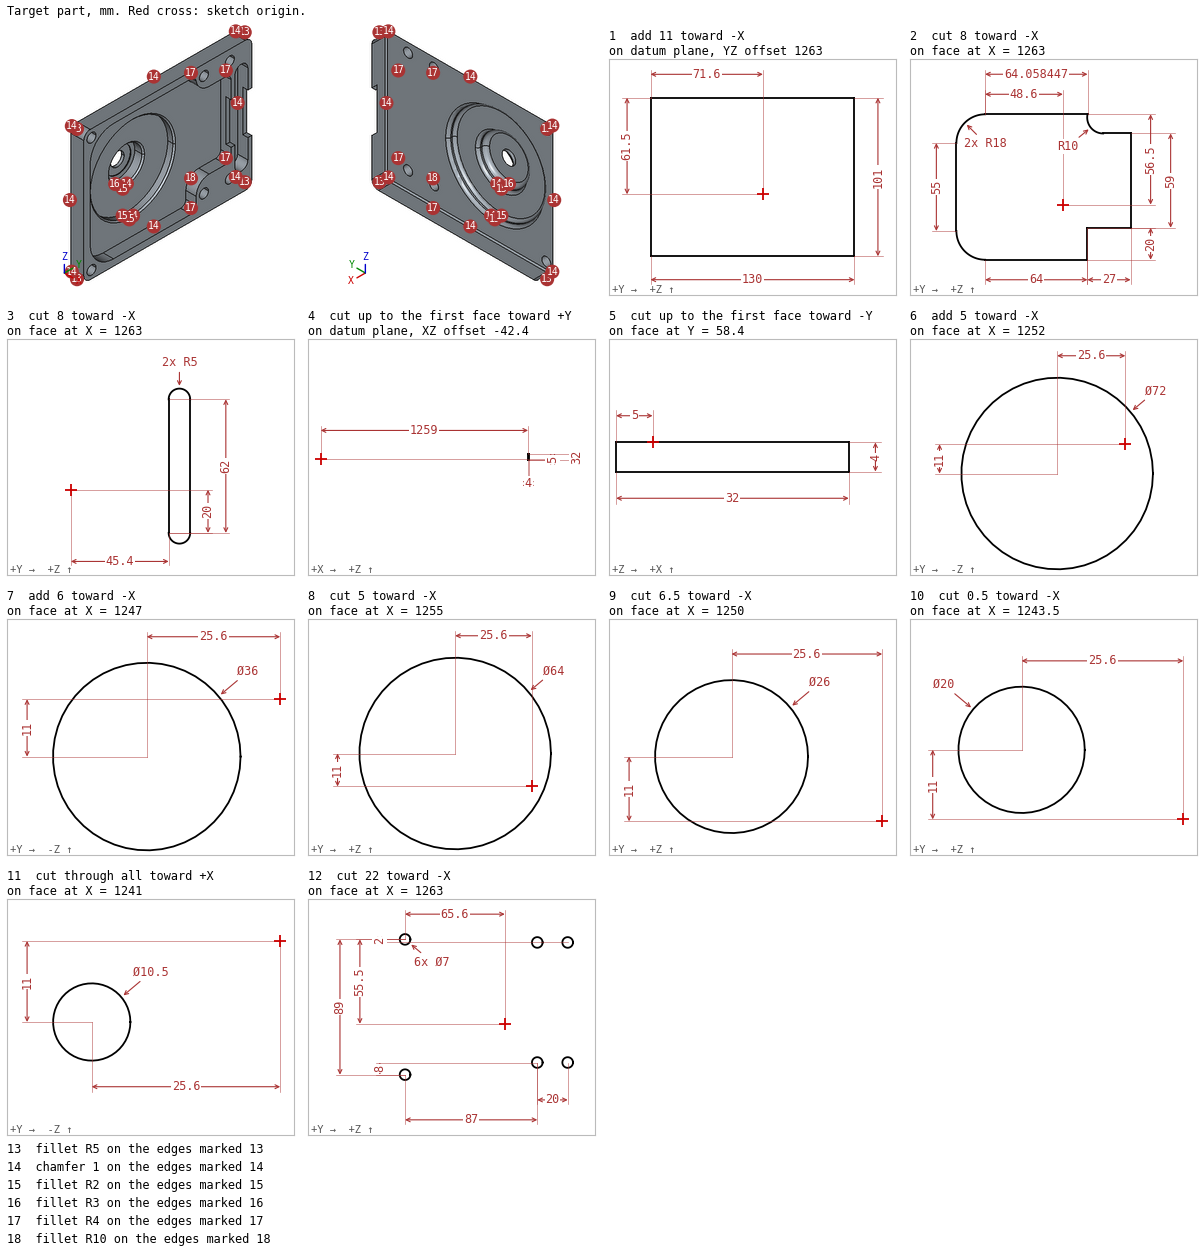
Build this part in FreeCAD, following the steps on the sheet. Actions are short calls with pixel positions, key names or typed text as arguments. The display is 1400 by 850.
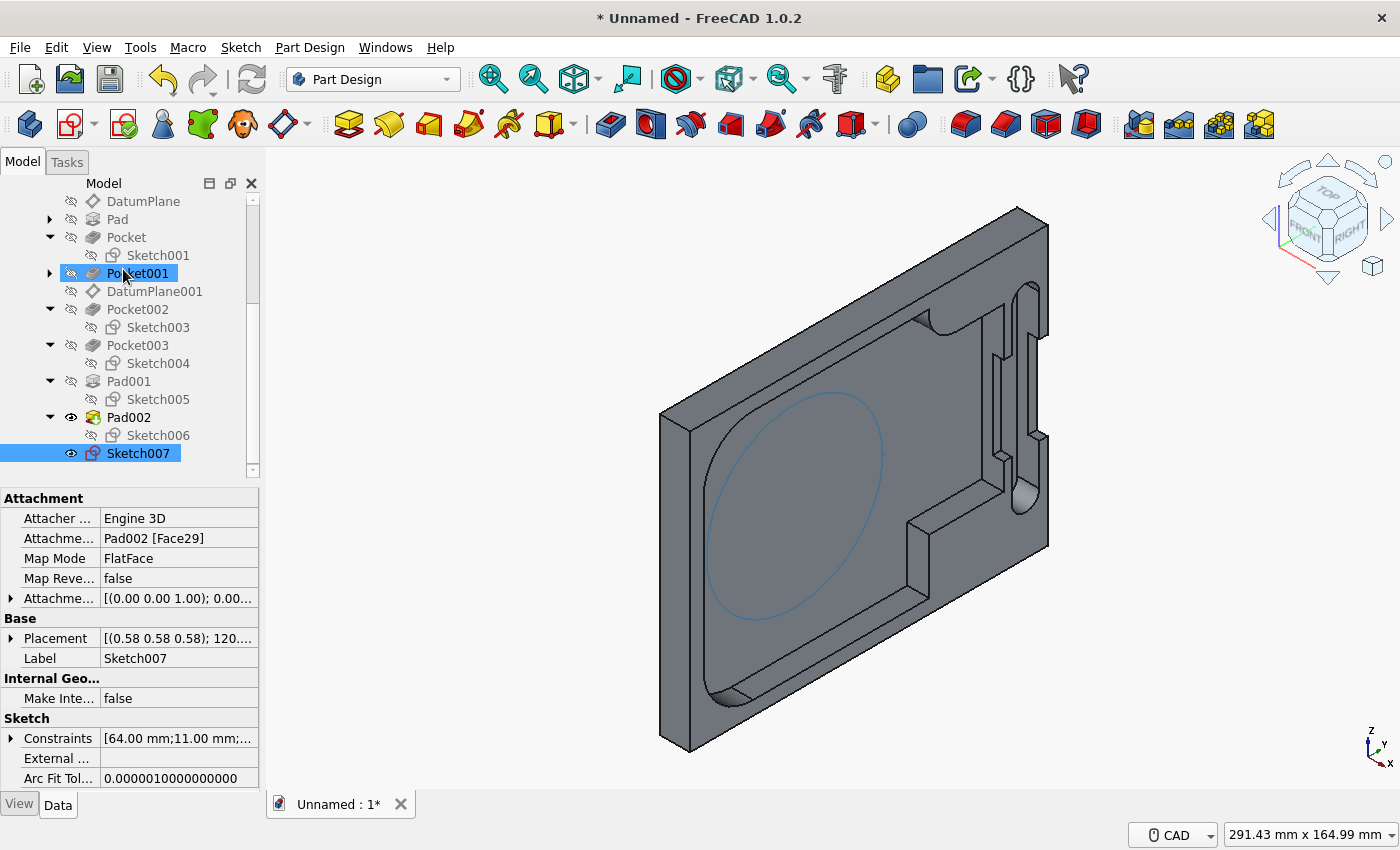
click(612, 124)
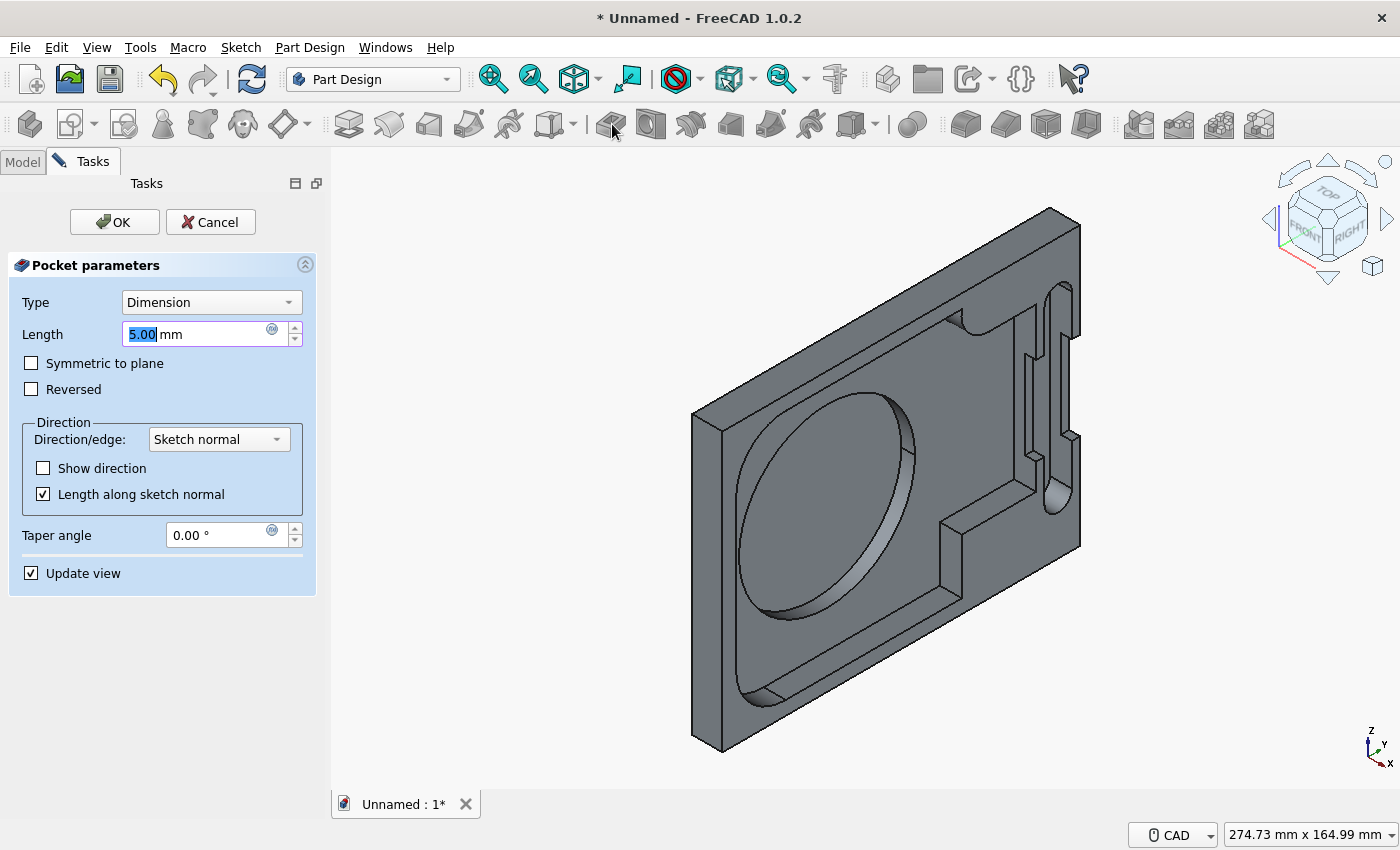
text(5)
key(Tab)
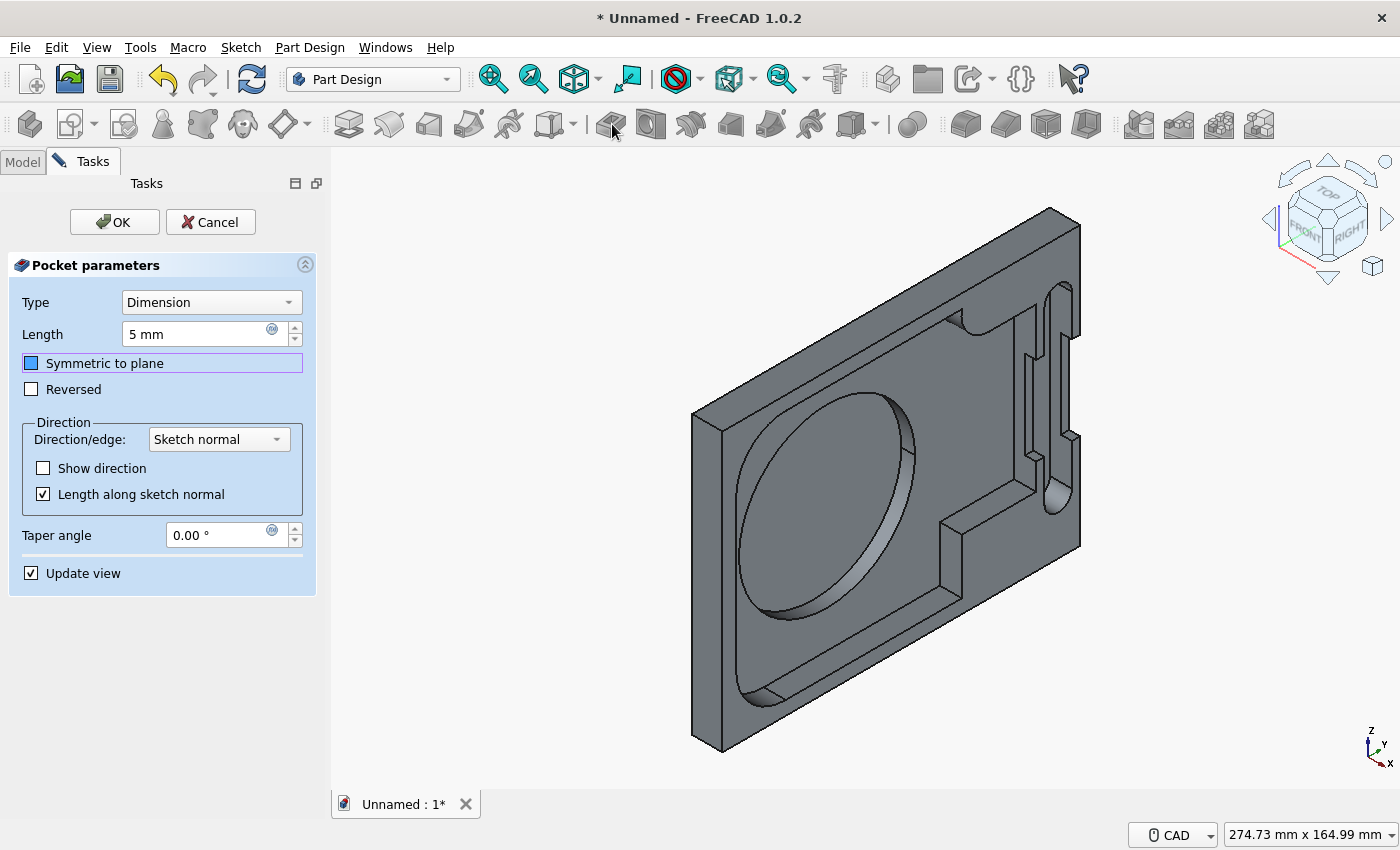
click(115, 222)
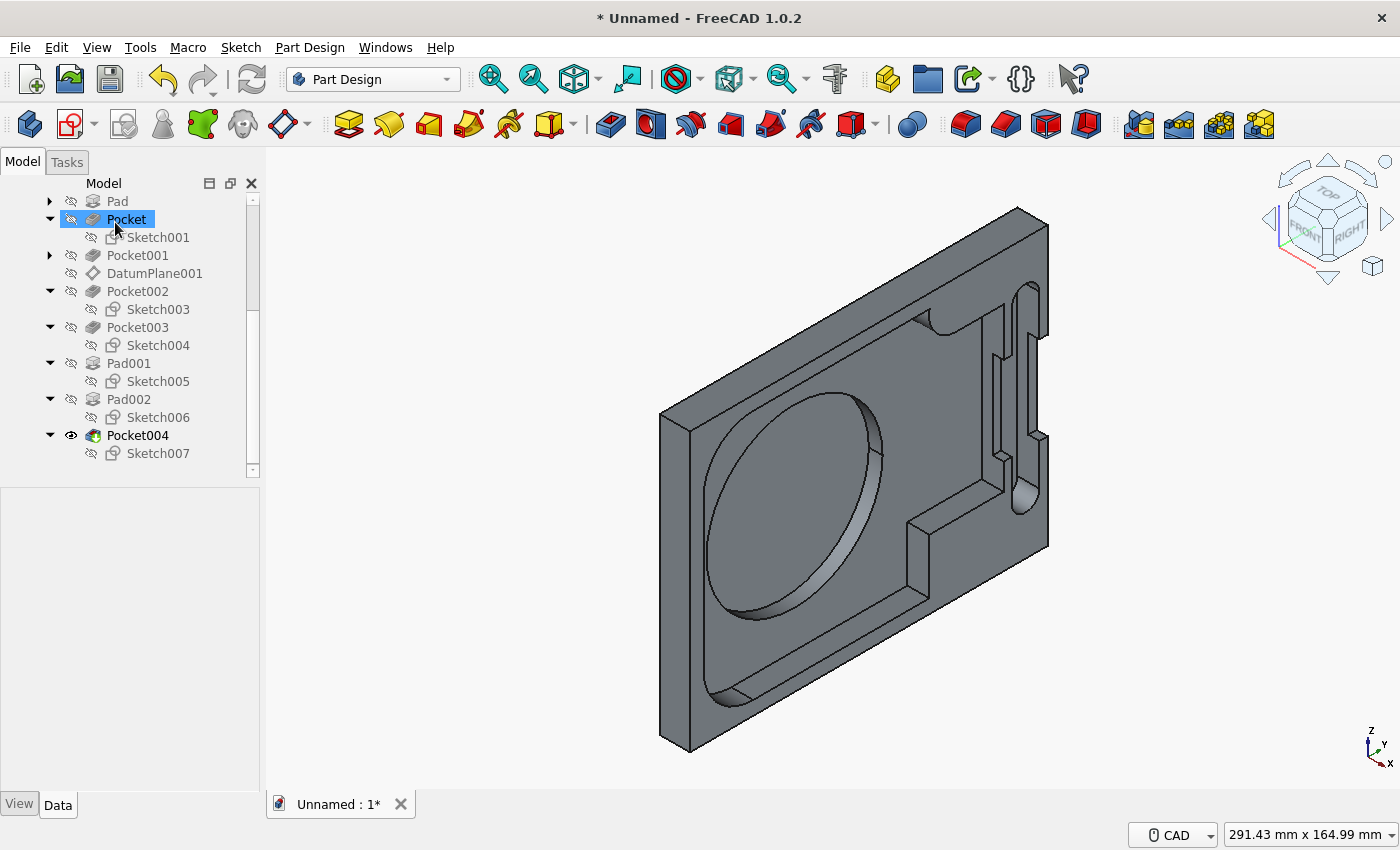
click(781, 497)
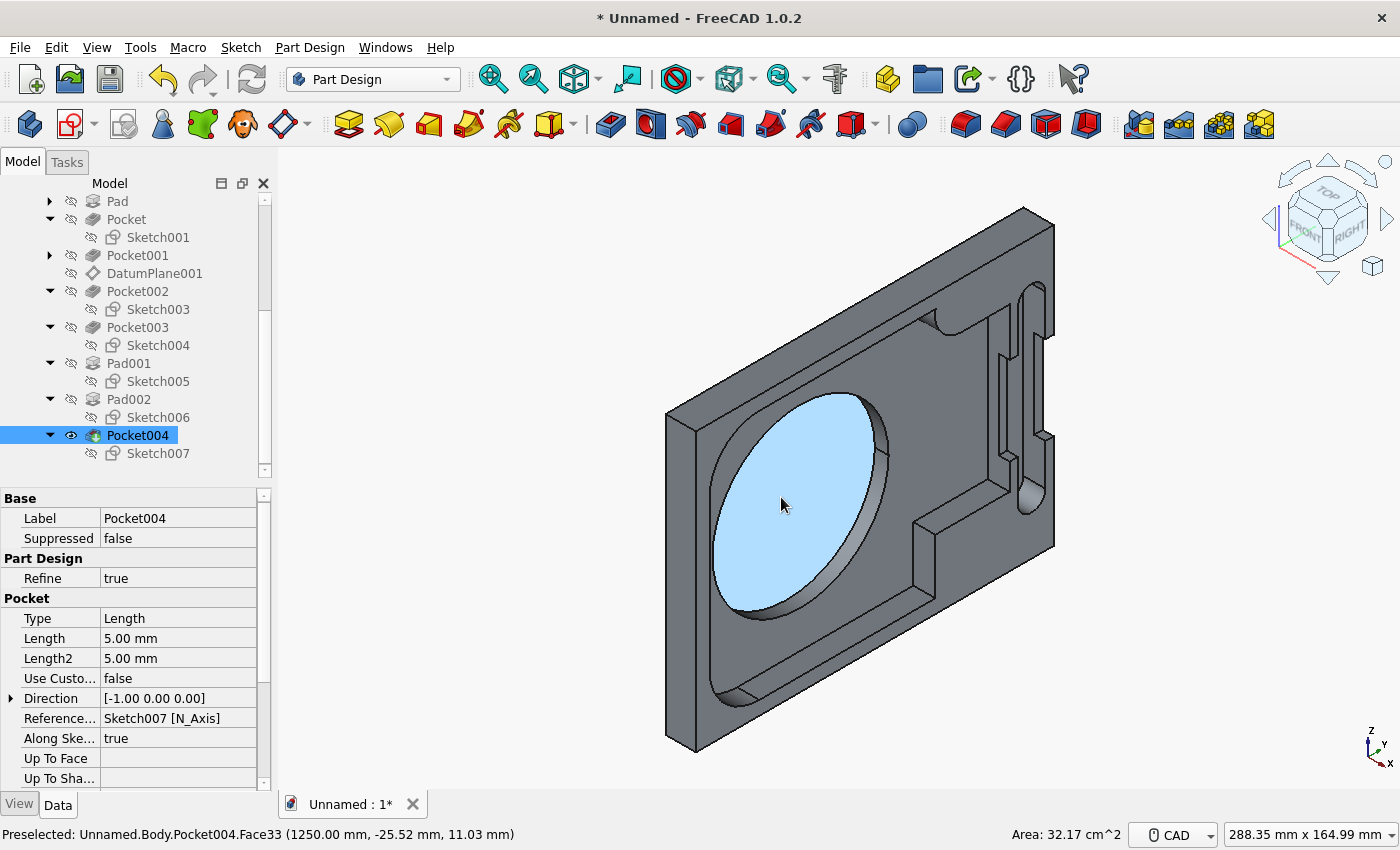
click(70, 124)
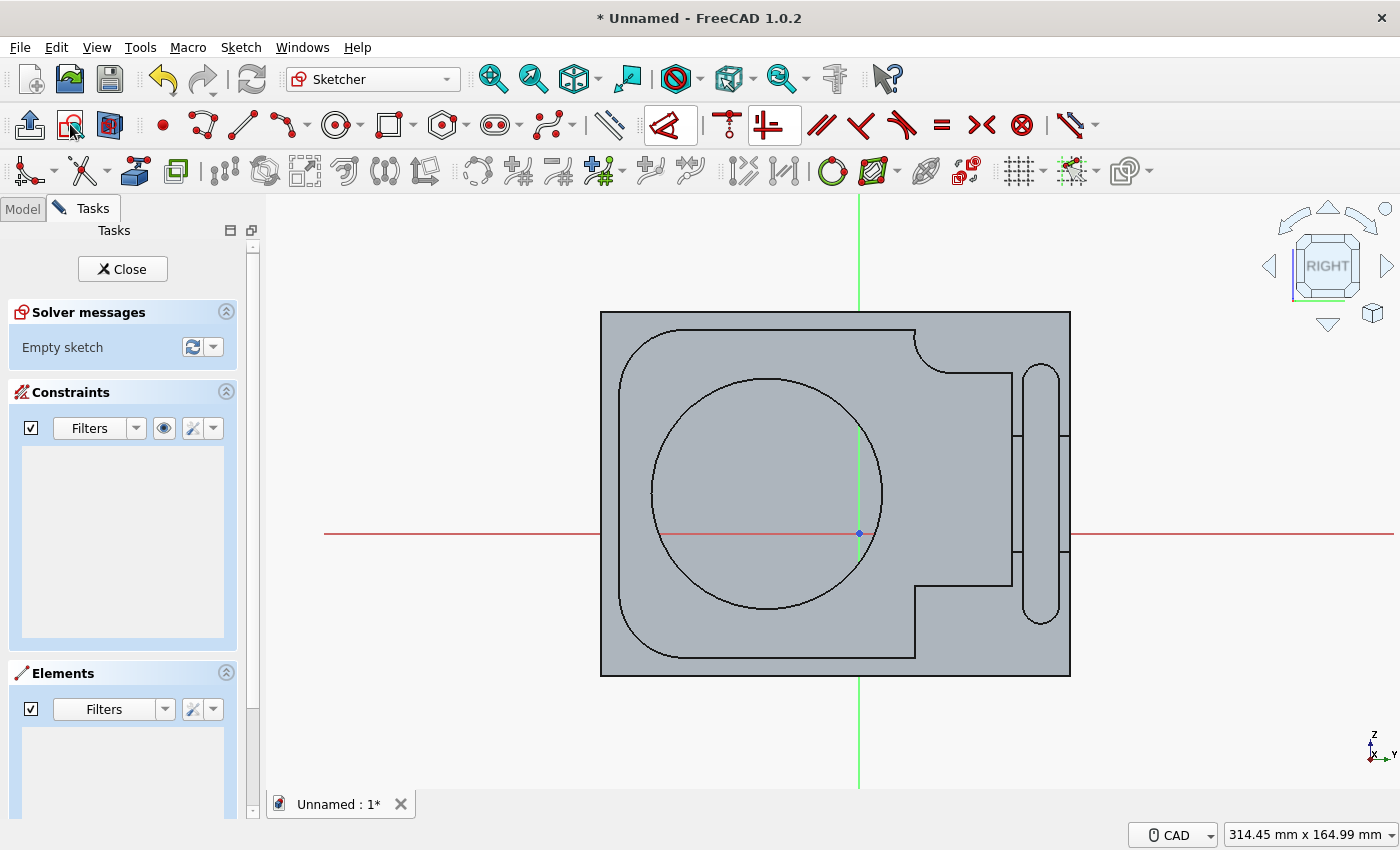
scroll(798, 495, up, 7)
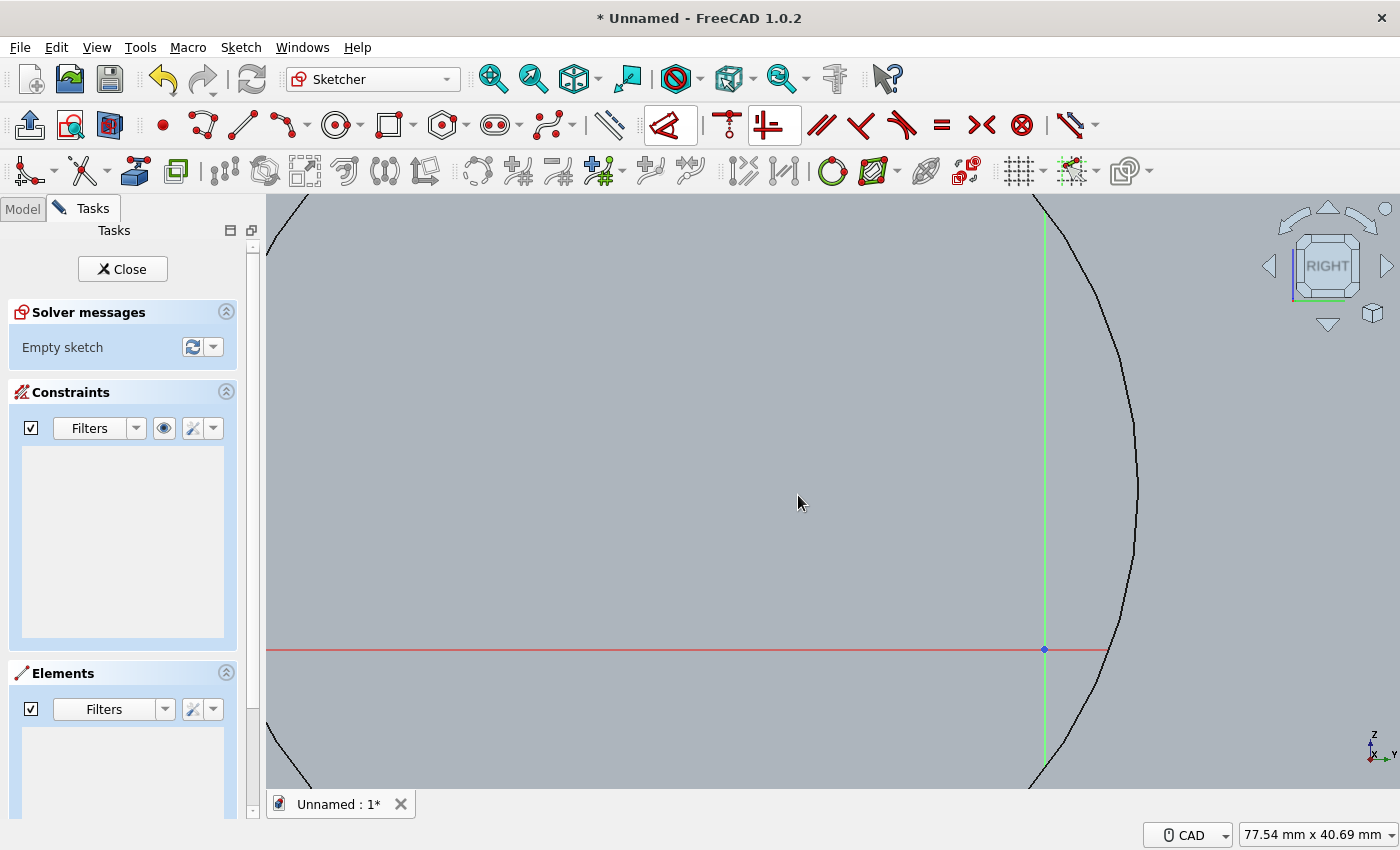
click(336, 126)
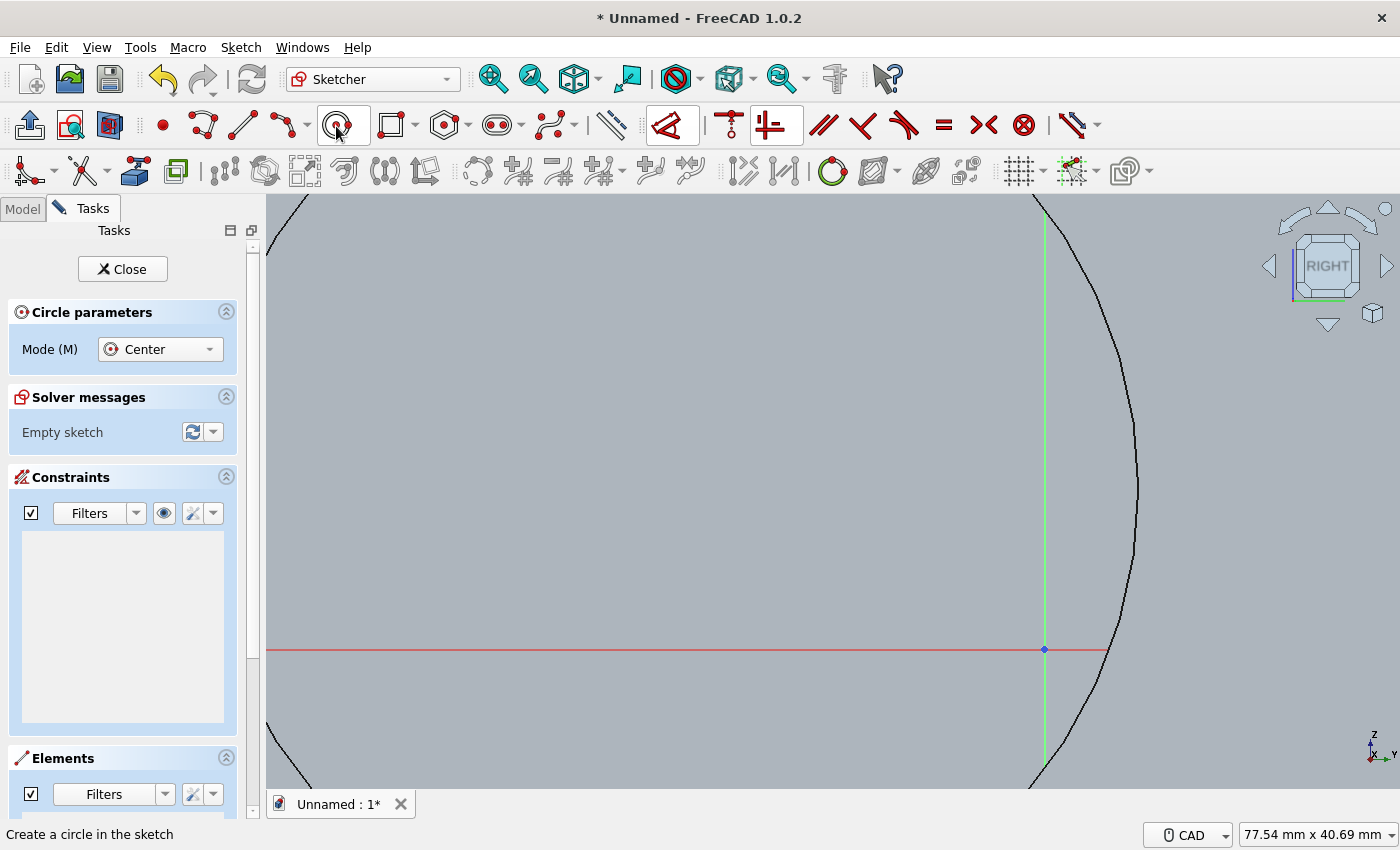
click(670, 489)
move(805, 355)